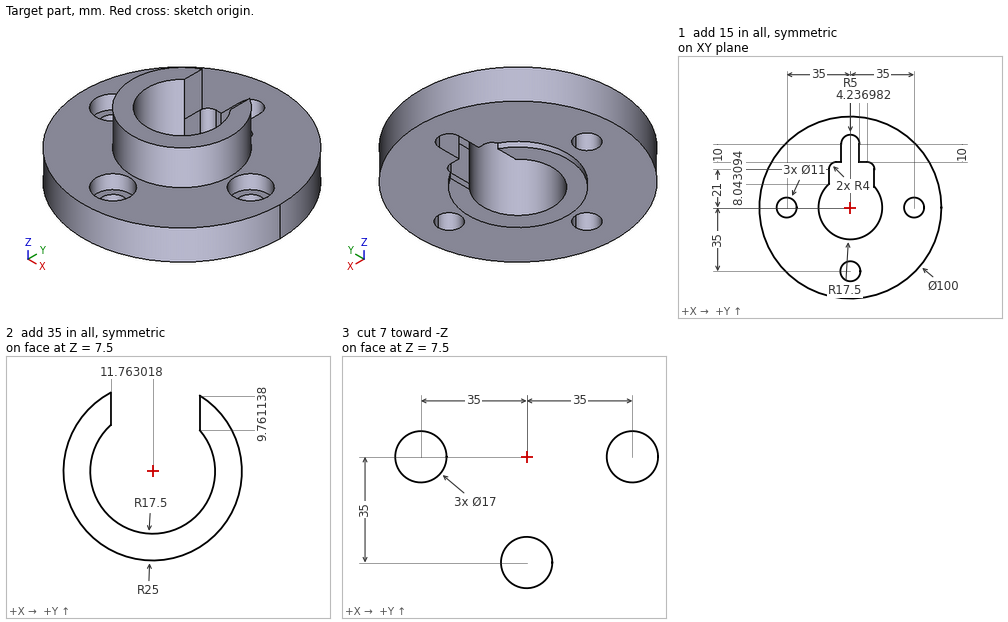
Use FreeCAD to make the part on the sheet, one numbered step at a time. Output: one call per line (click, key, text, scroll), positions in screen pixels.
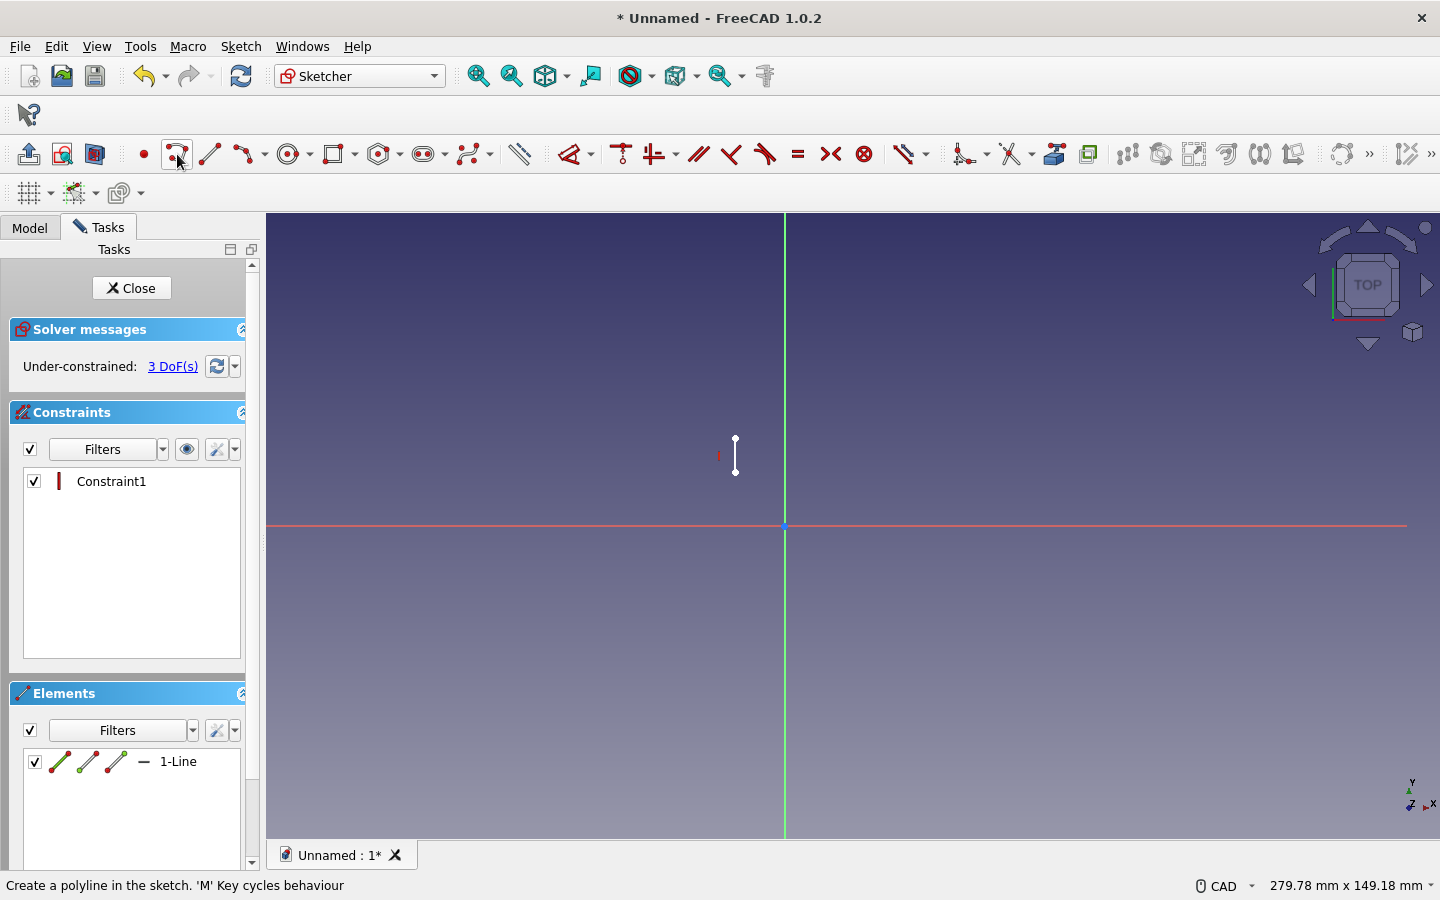
click(752, 421)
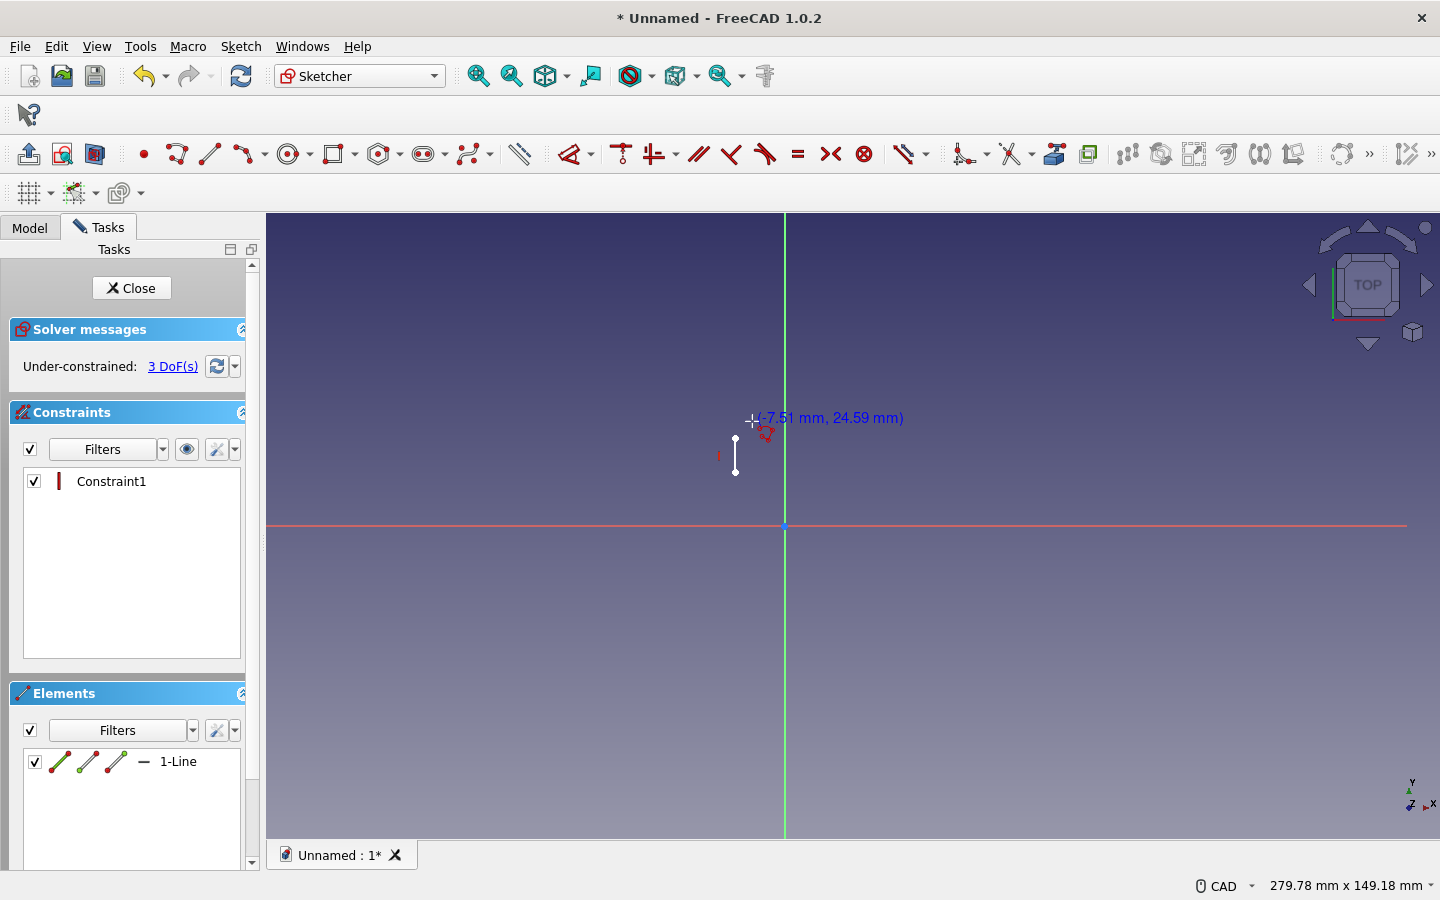
scroll(764, 421, up, 2)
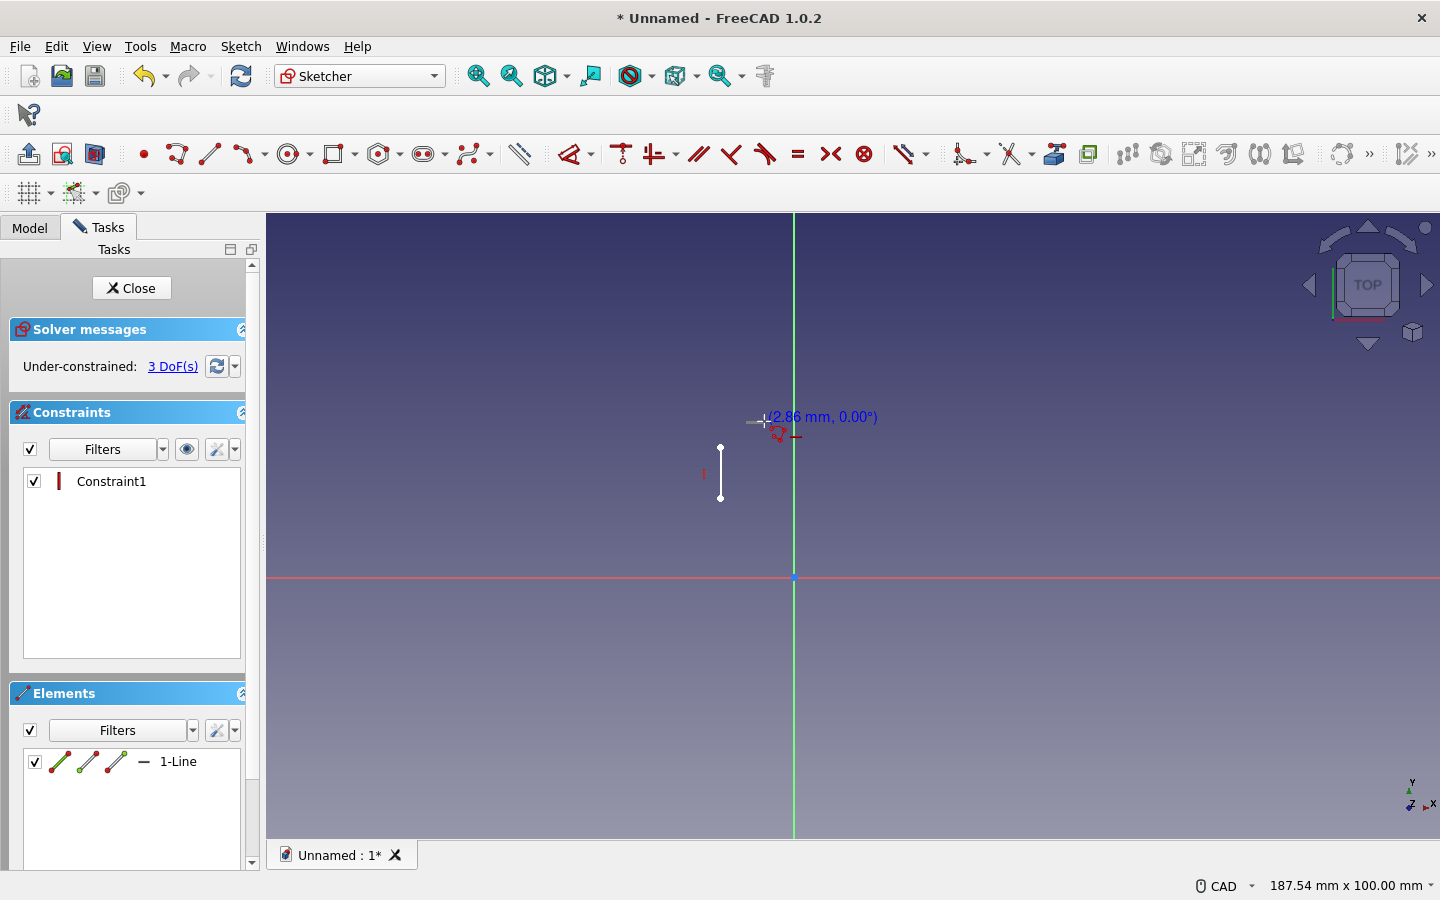
click(763, 421)
click(763, 359)
right_click(763, 359)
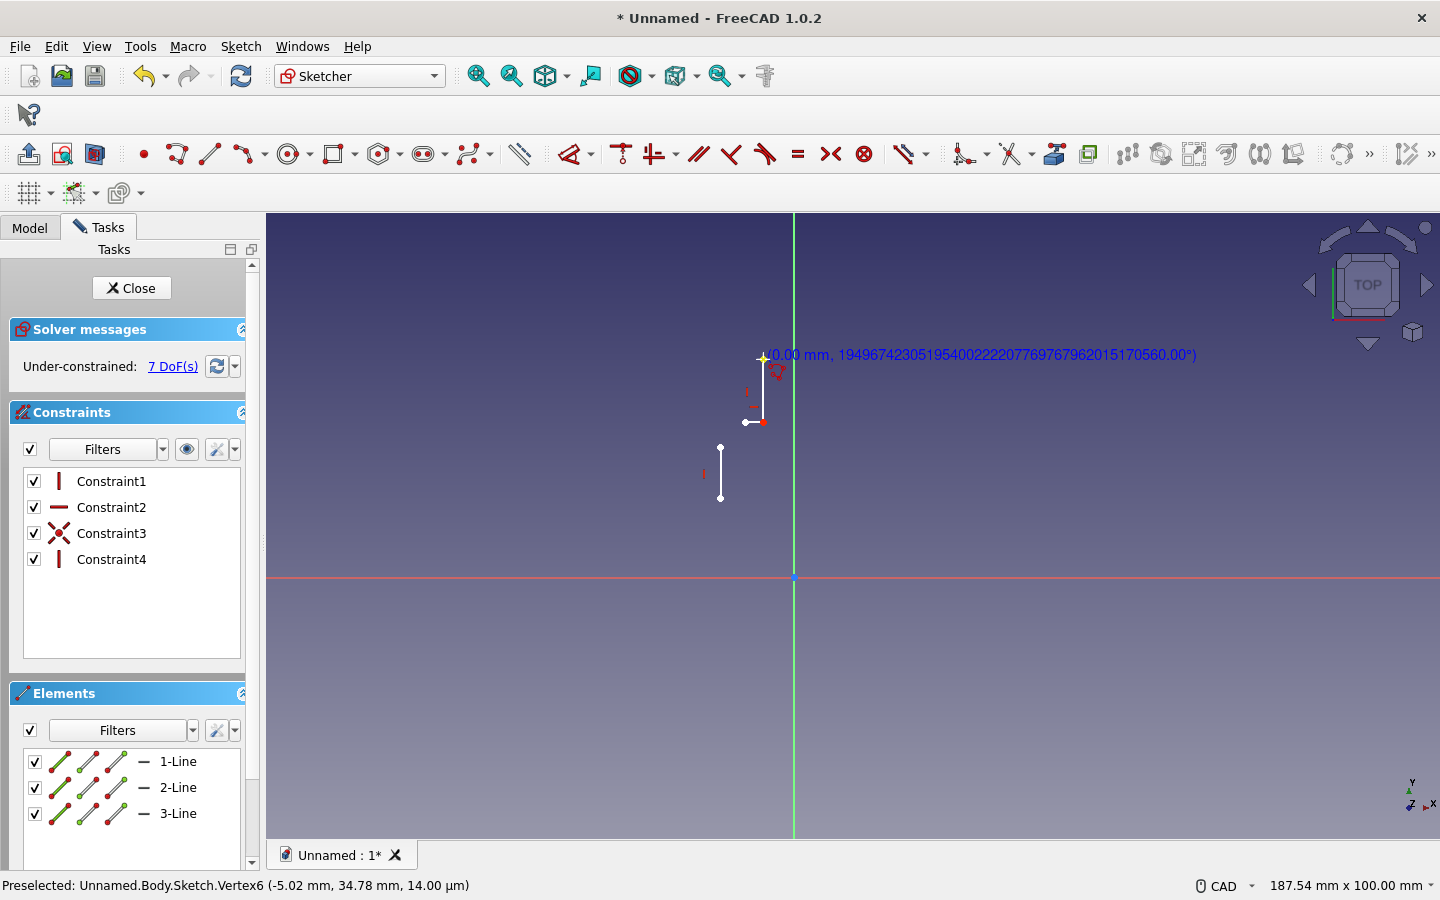
click(826, 359)
click(826, 421)
click(852, 421)
right_click(852, 421)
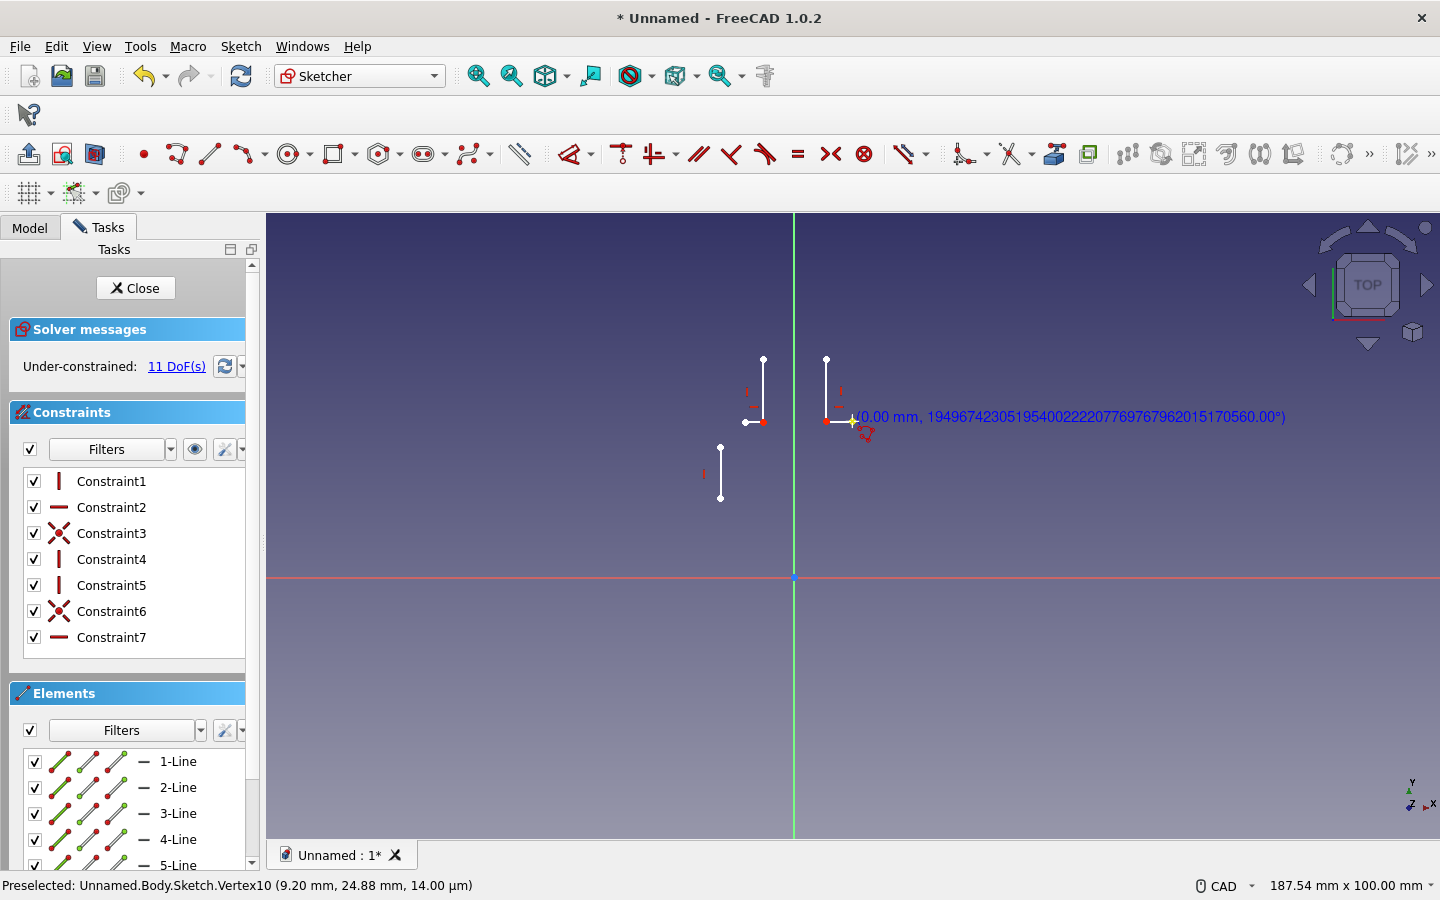
key(g)
key(l)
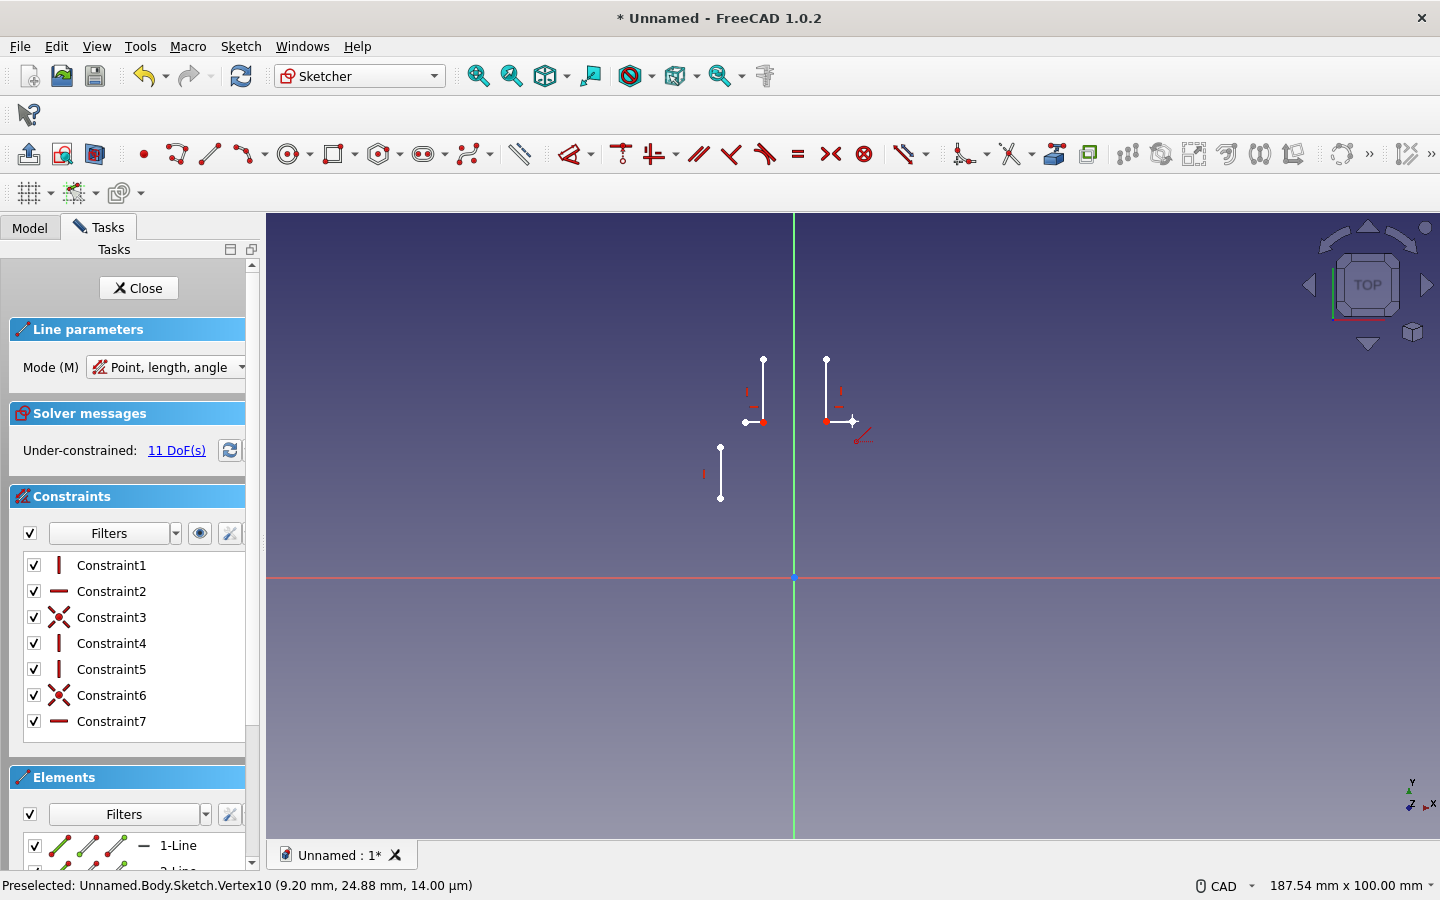
click(877, 446)
click(877, 506)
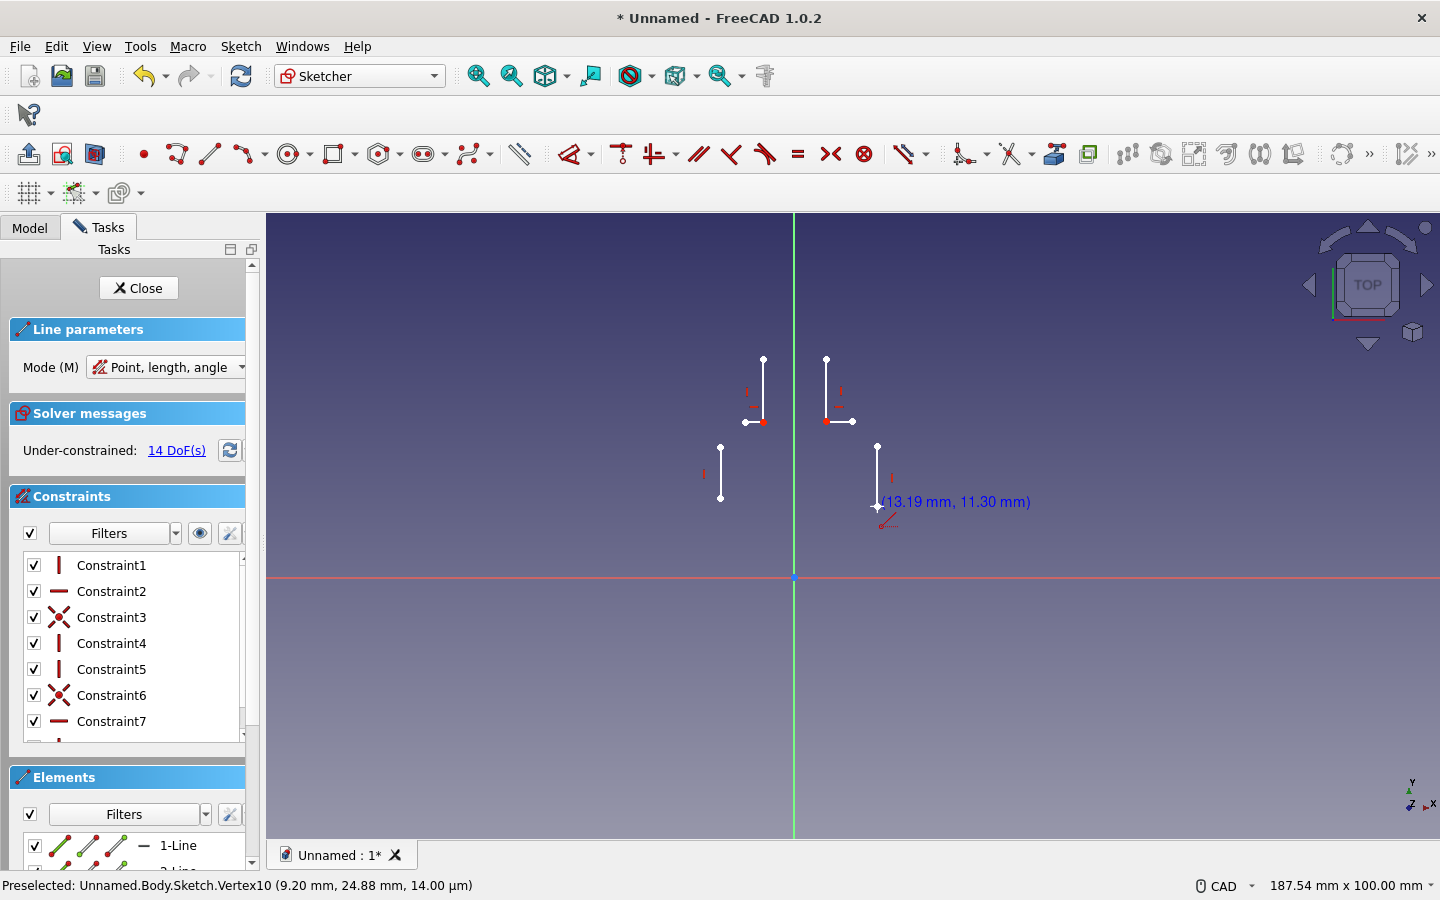
click(242, 154)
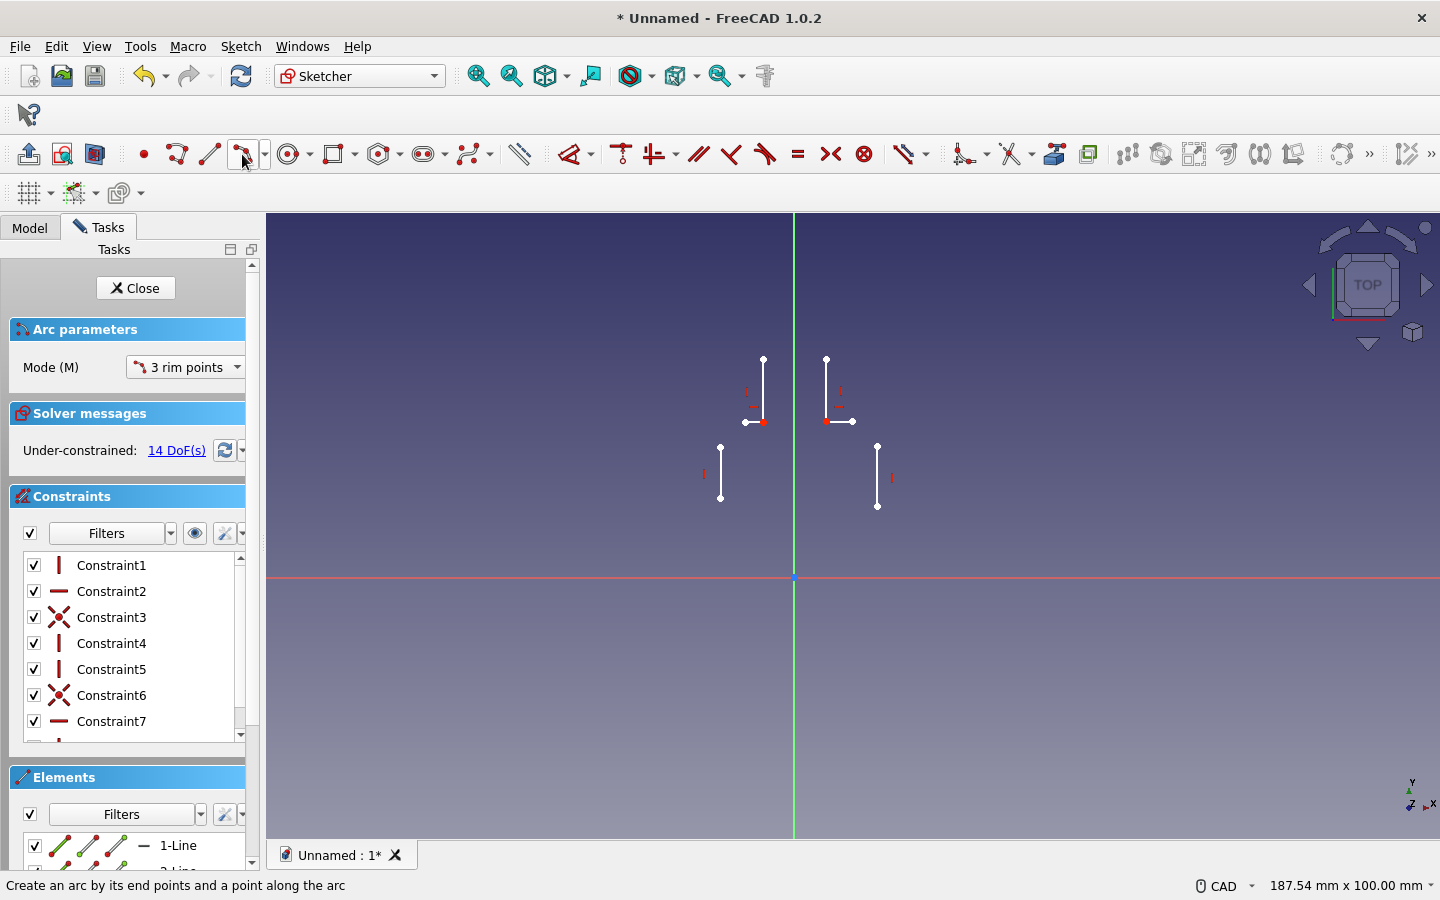
click(721, 448)